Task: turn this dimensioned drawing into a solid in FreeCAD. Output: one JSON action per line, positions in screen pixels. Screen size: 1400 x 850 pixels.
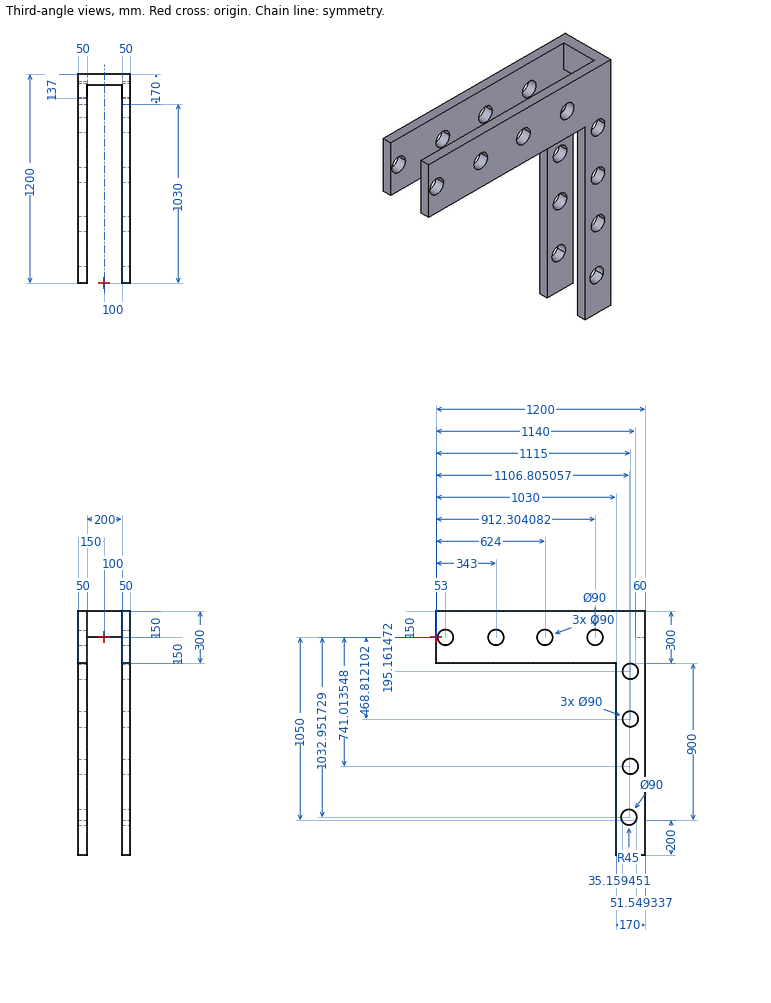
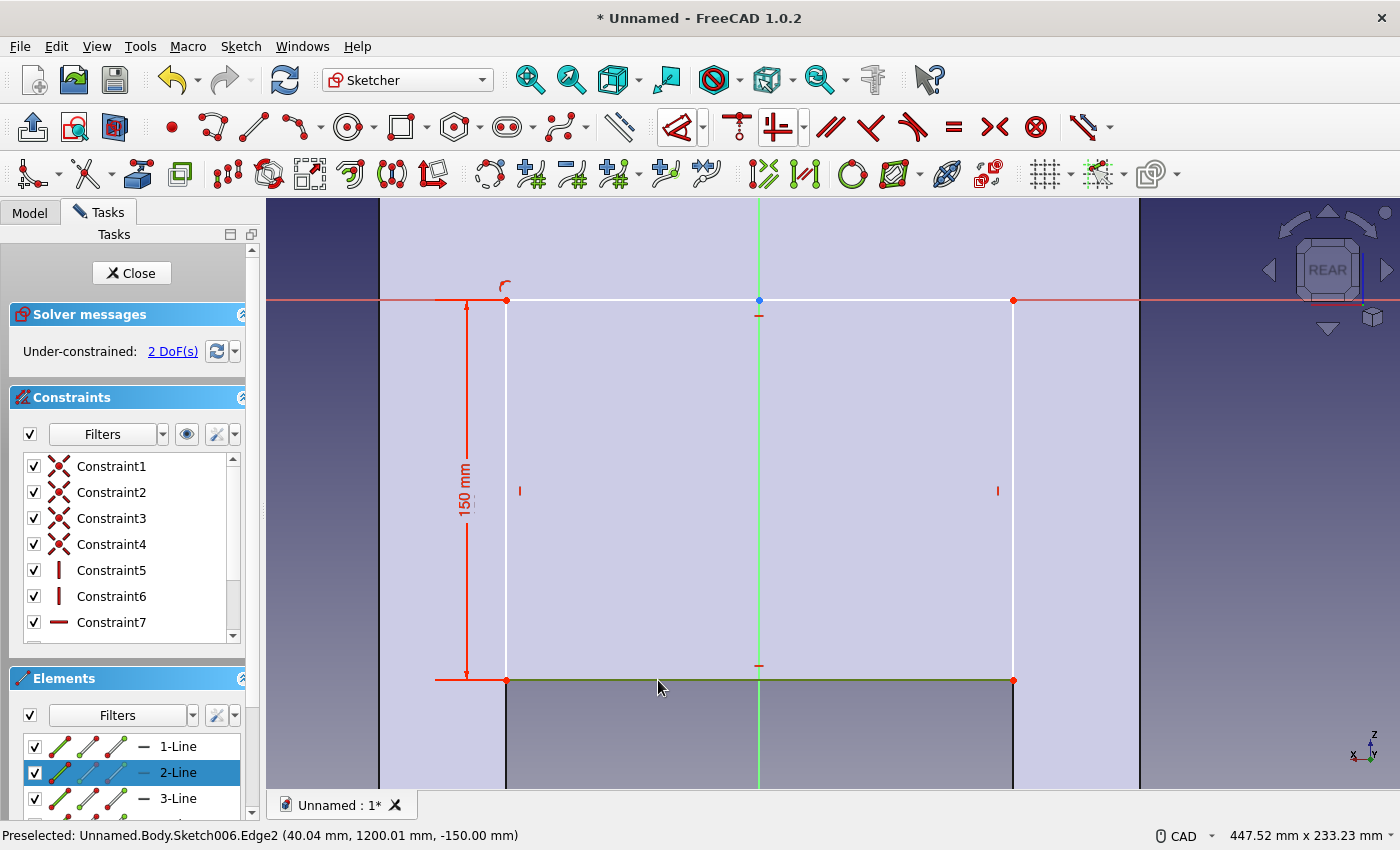
{"action": "left_click", "coordinate": [702, 128]}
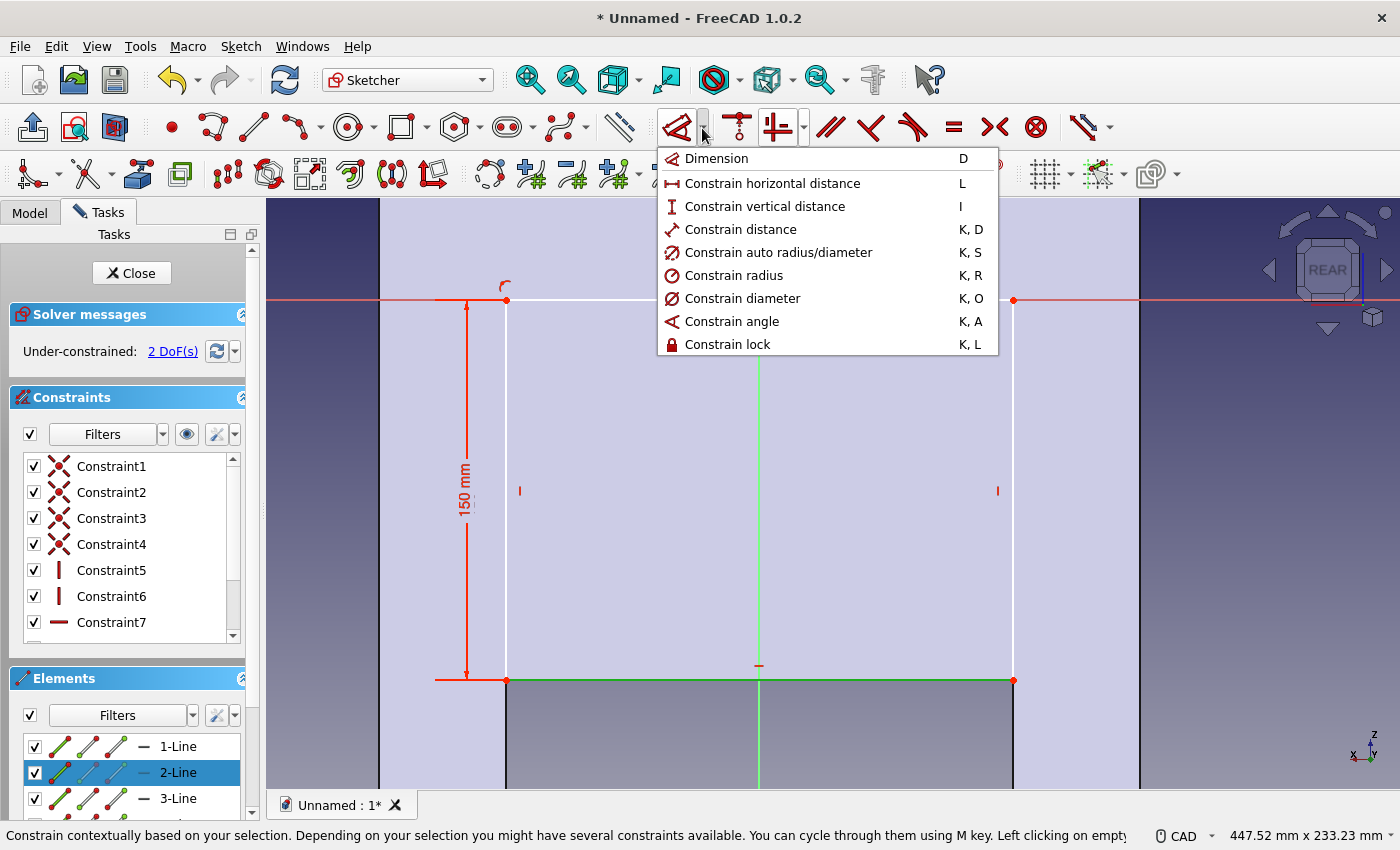
{"action": "left_click", "coordinate": [828, 184]}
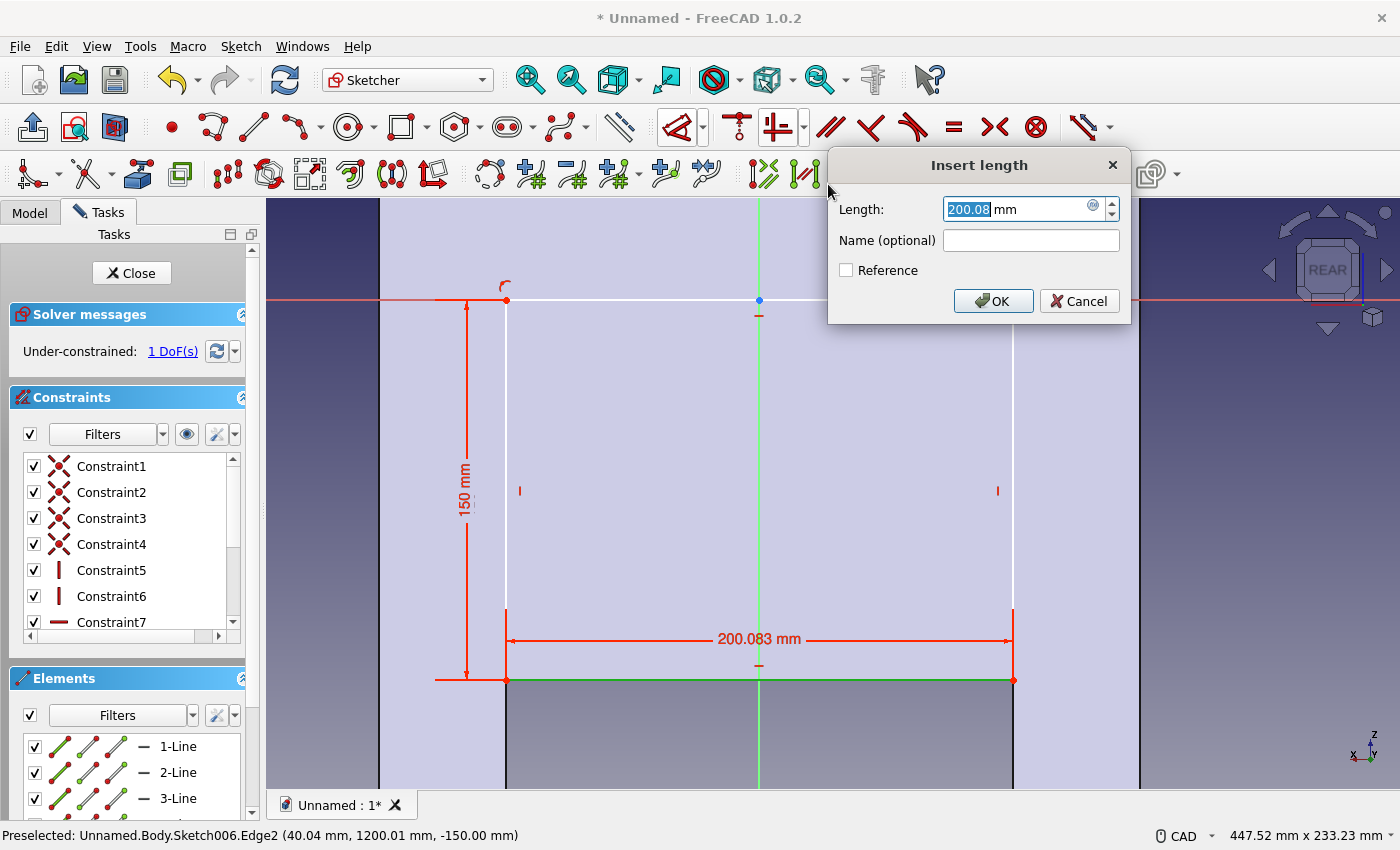
{"action": "type", "text": "200"}
{"action": "key", "text": "Return"}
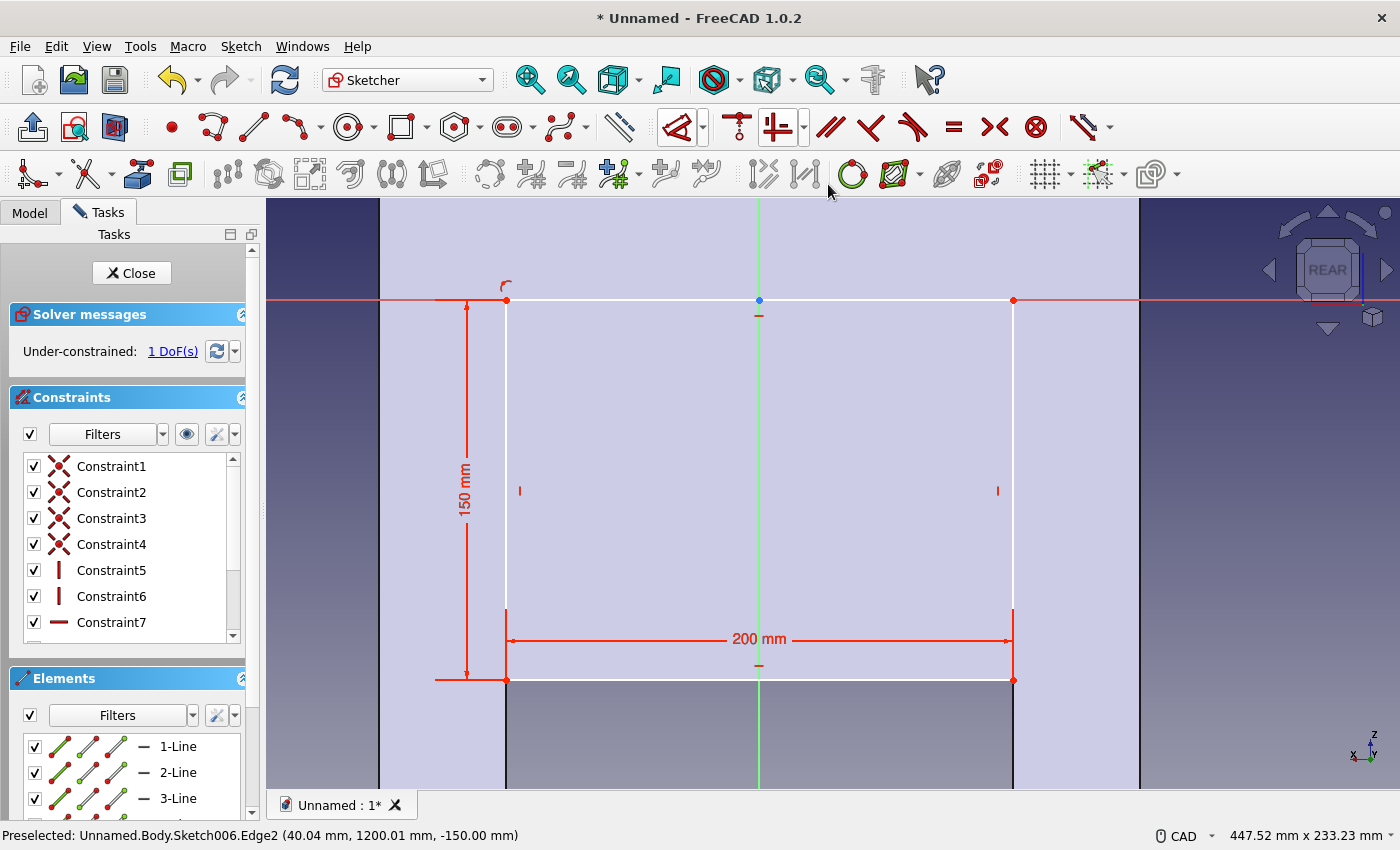
{"action": "left_click", "coordinate": [506, 300]}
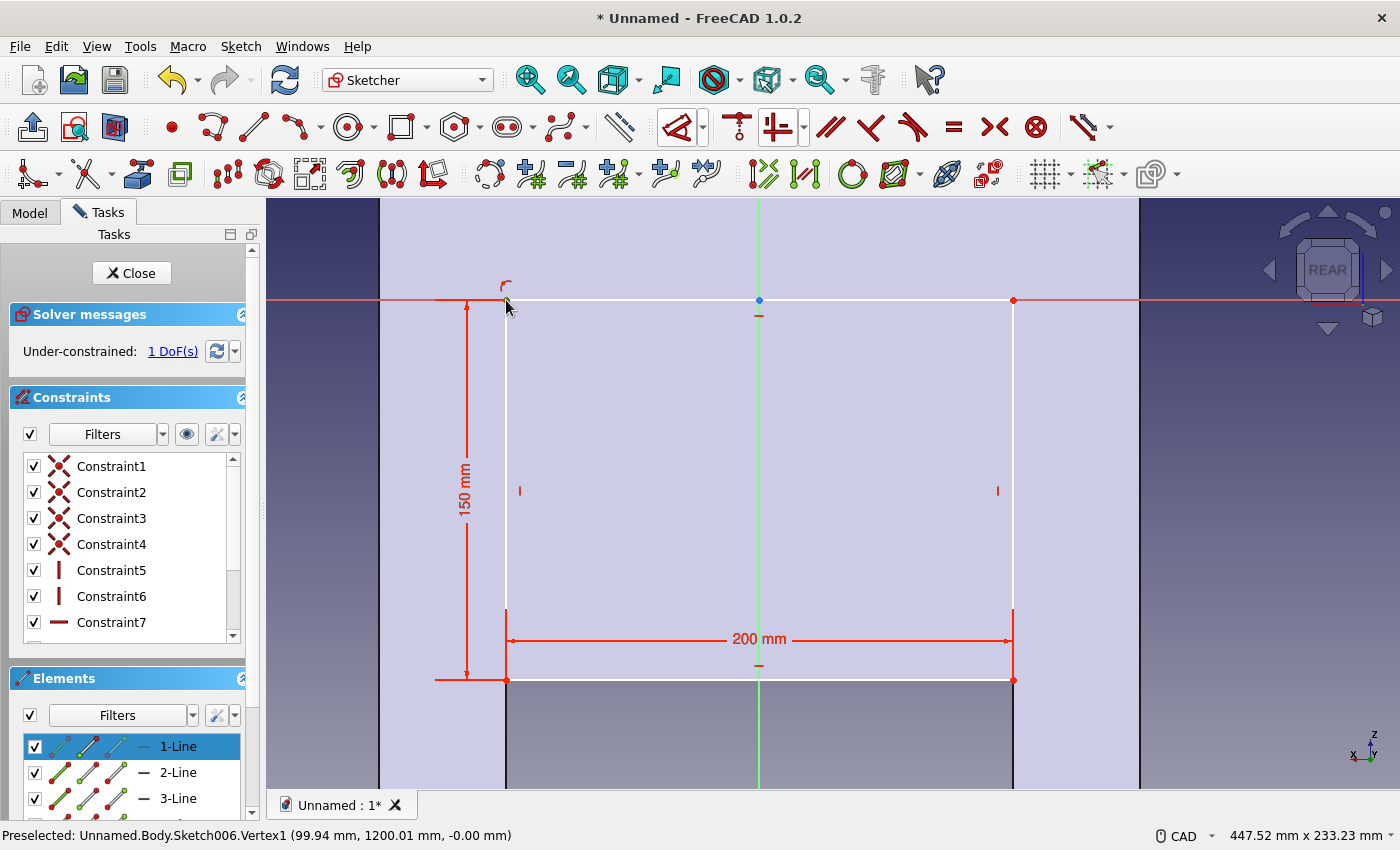
{"action": "left_click", "coordinate": [702, 128]}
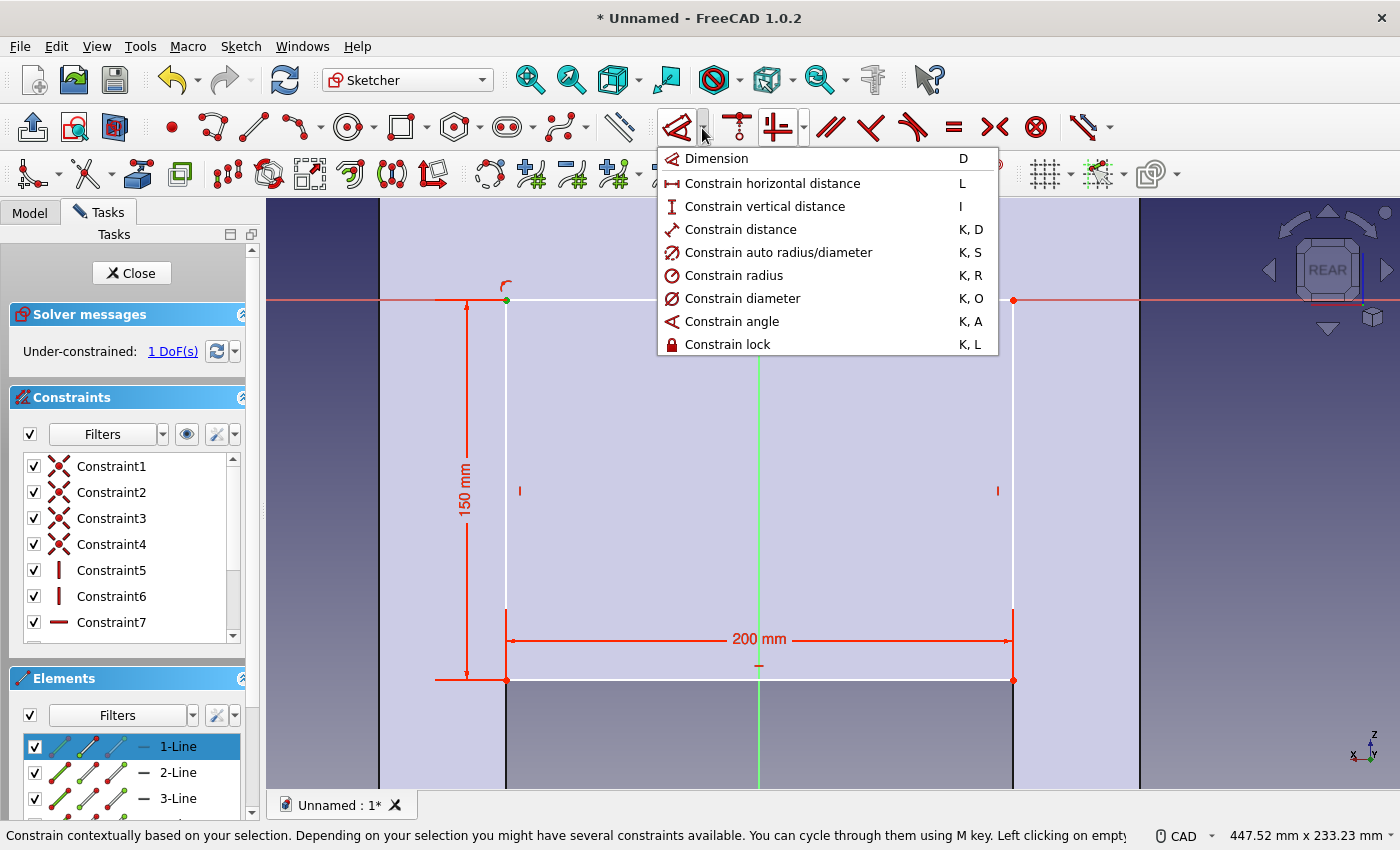
{"action": "left_click", "coordinate": [828, 184]}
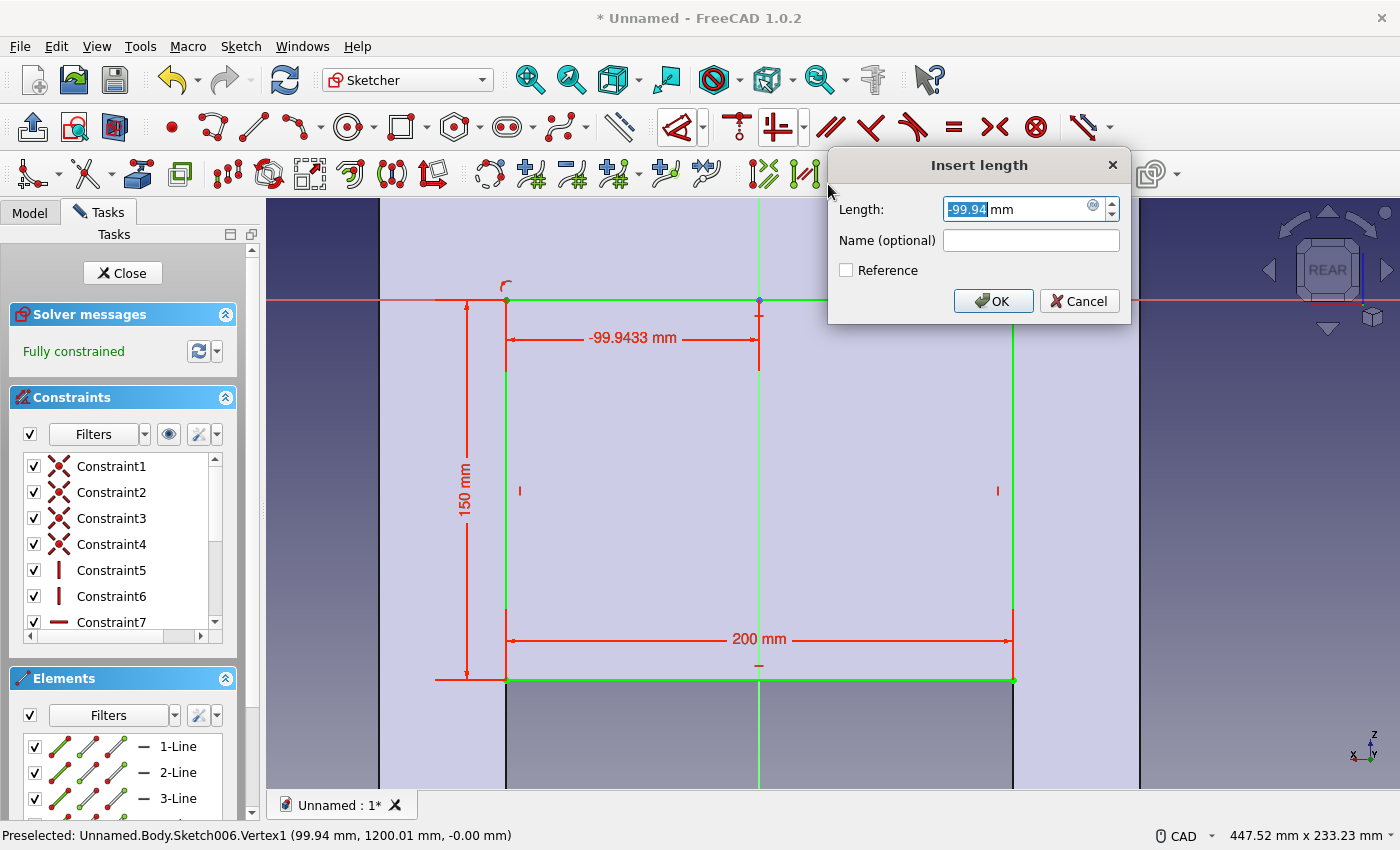
{"action": "type", "text": "-100"}
{"action": "key", "text": "Return"}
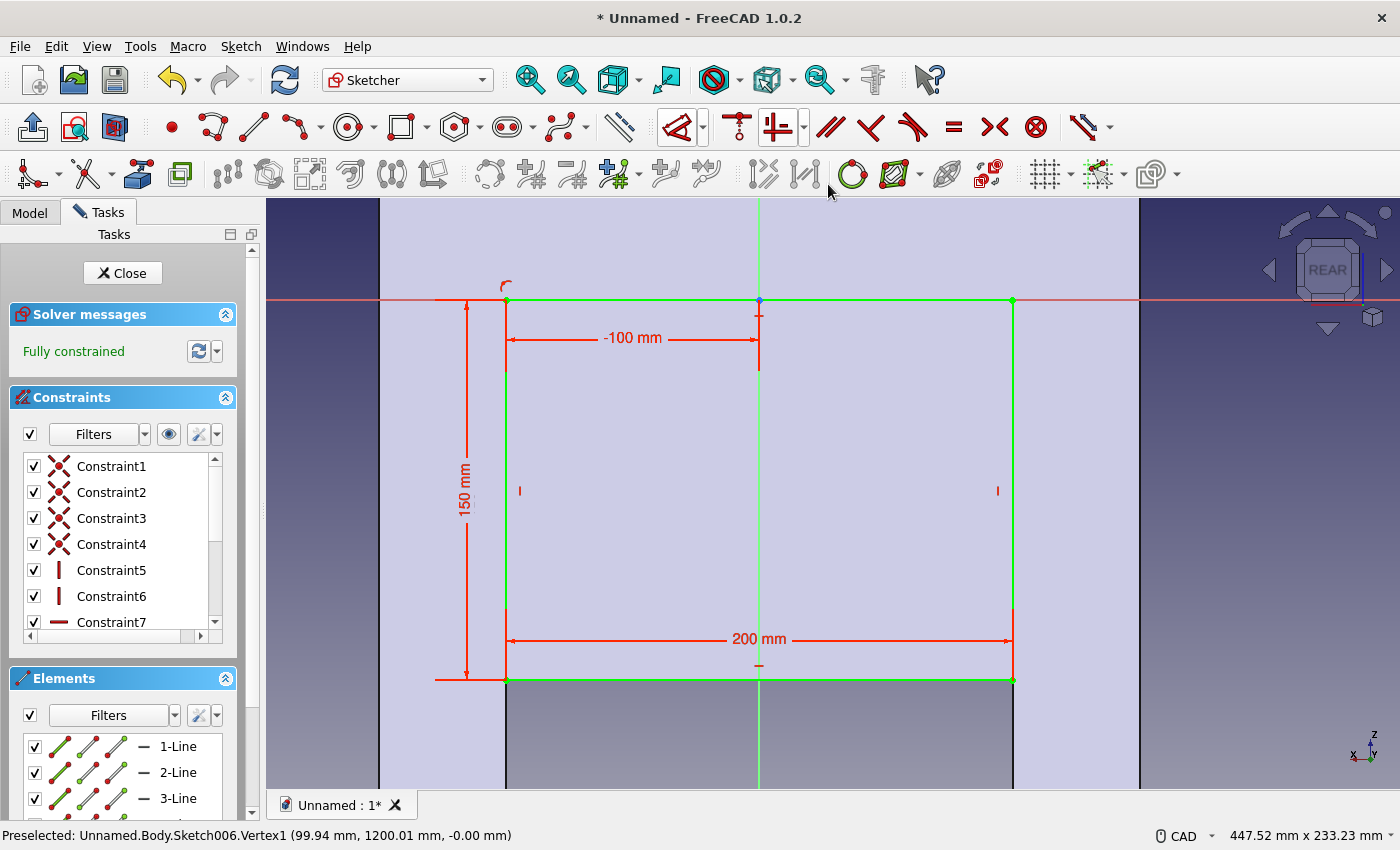
{"action": "left_click", "coordinate": [123, 273]}